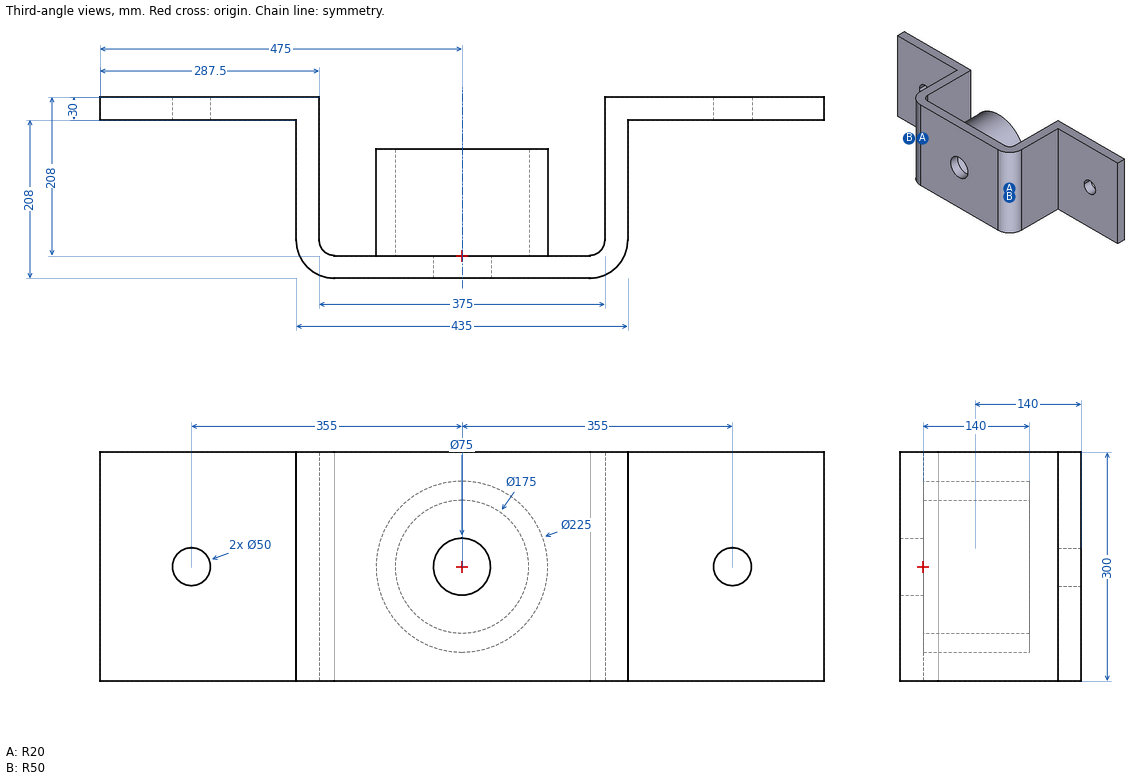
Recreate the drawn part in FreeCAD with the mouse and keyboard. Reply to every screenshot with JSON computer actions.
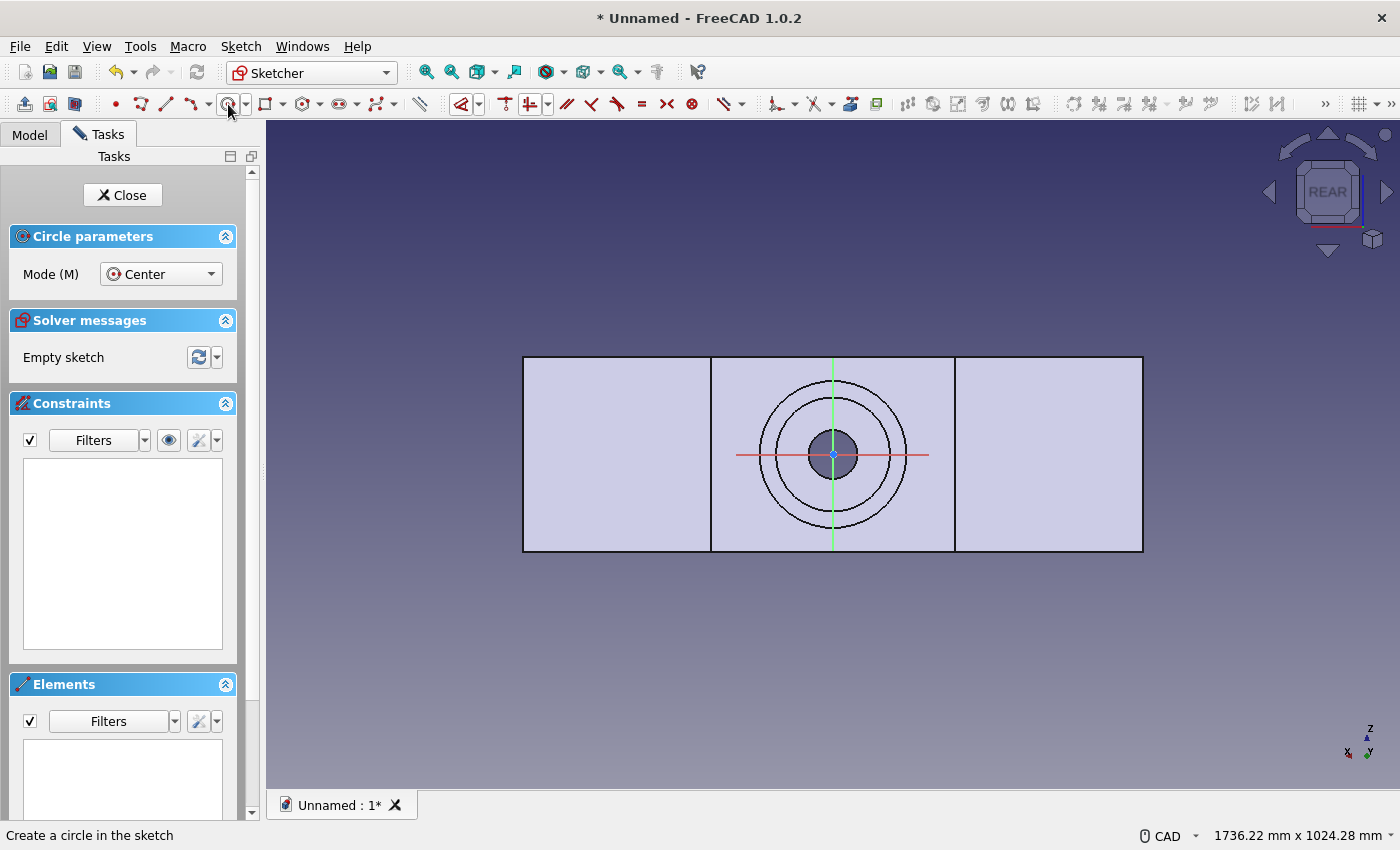
{"action": "scroll", "coordinate": [1065, 455], "scroll_direction": "up", "scroll_amount": 2}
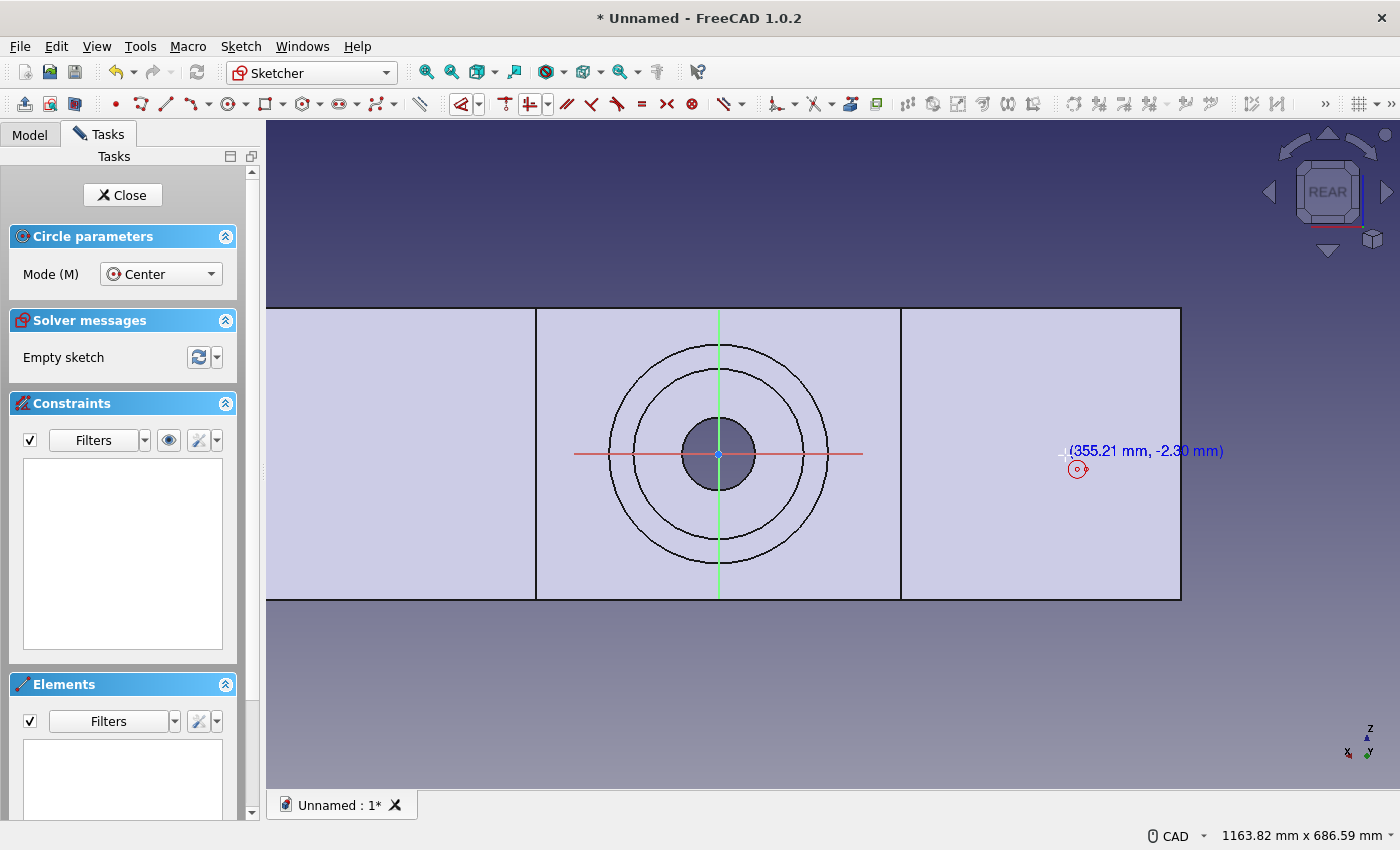
{"action": "left_click", "coordinate": [1064, 454]}
{"action": "mouse_move", "coordinate": [1082, 437]}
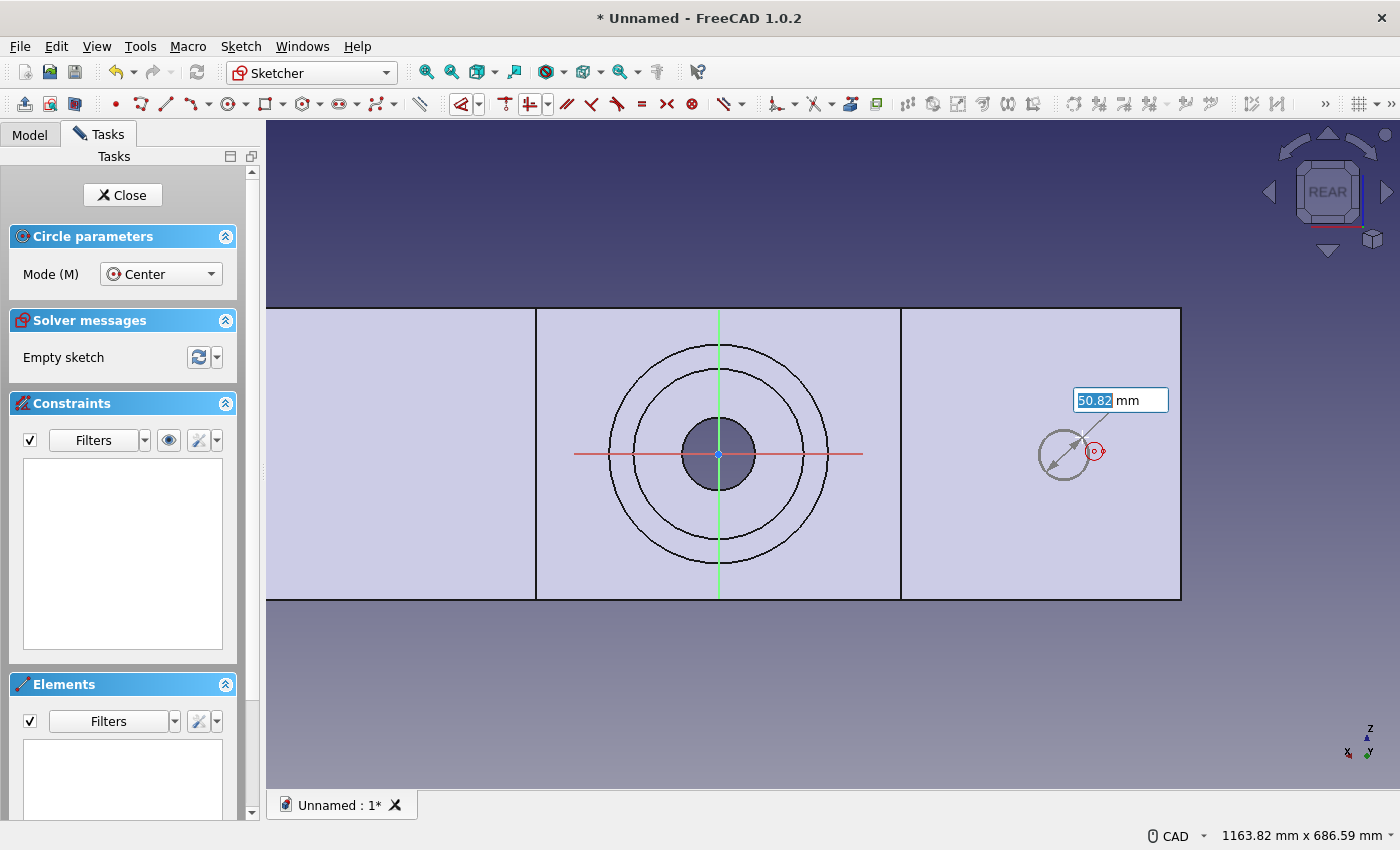
{"action": "type", "text": "50"}
{"action": "key", "text": "Return"}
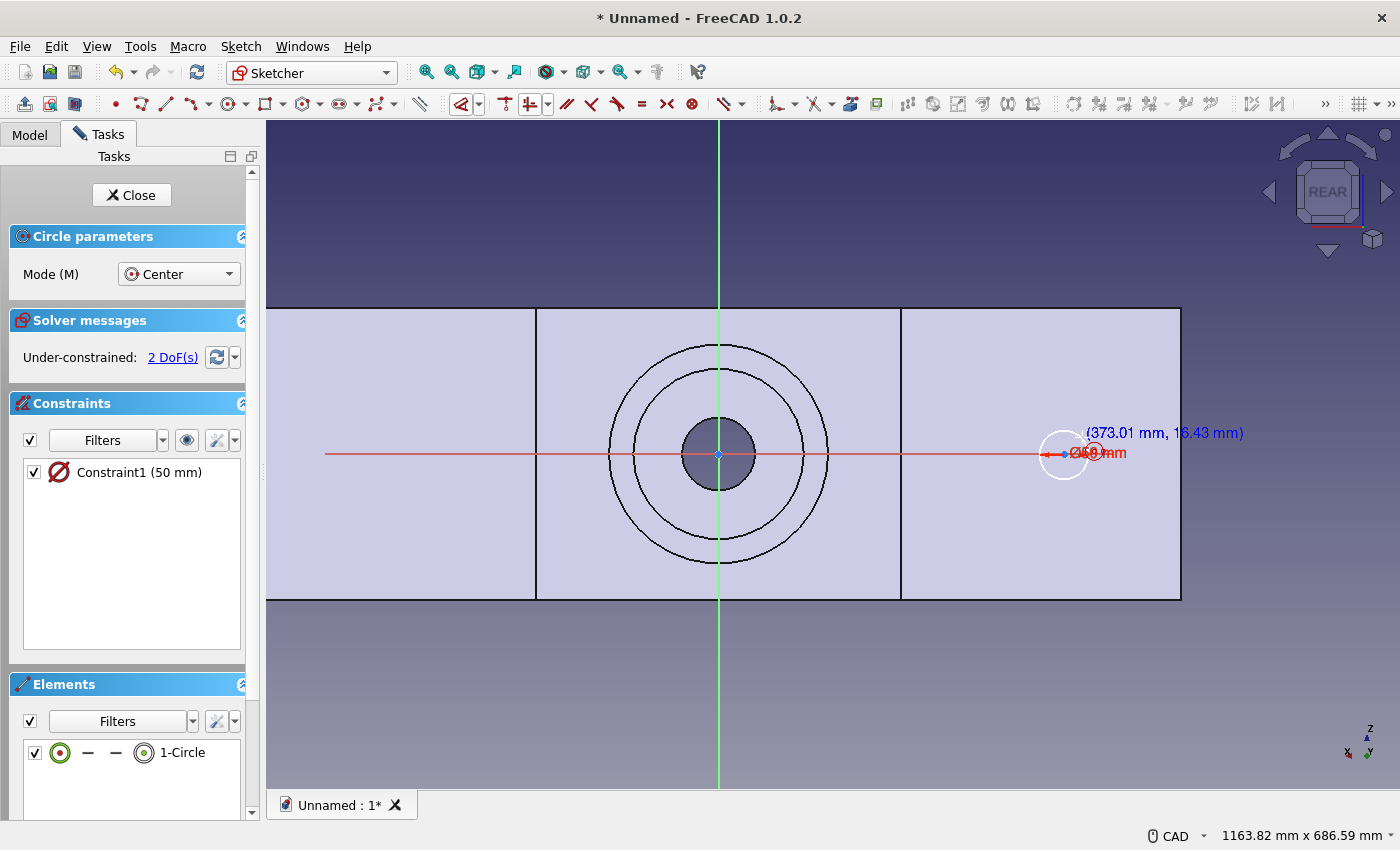
{"action": "left_click", "coordinate": [373, 454]}
{"action": "mouse_move", "coordinate": [390, 437]}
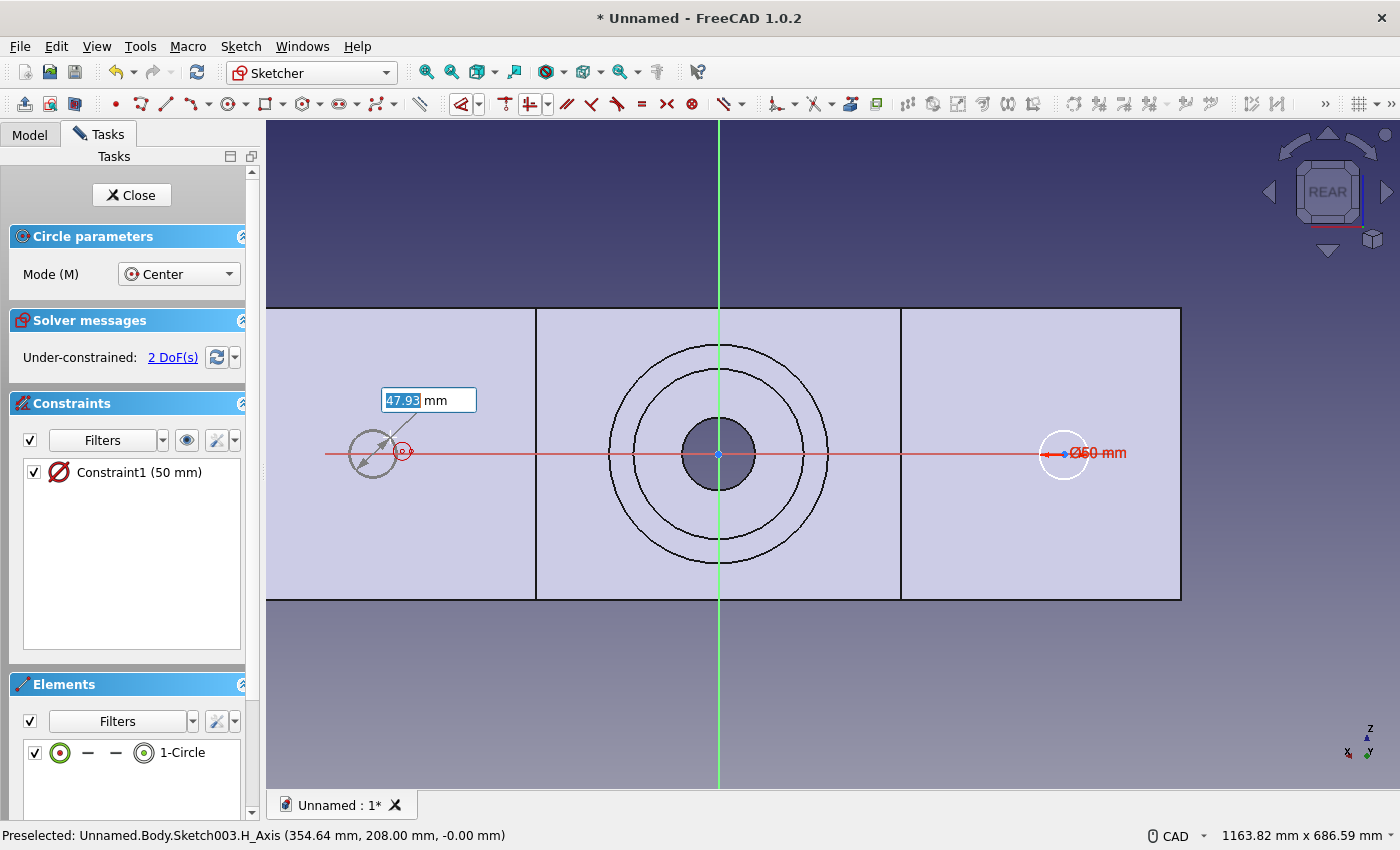
{"action": "type", "text": "50"}
{"action": "key", "text": "Return"}
{"action": "key", "text": "Escape"}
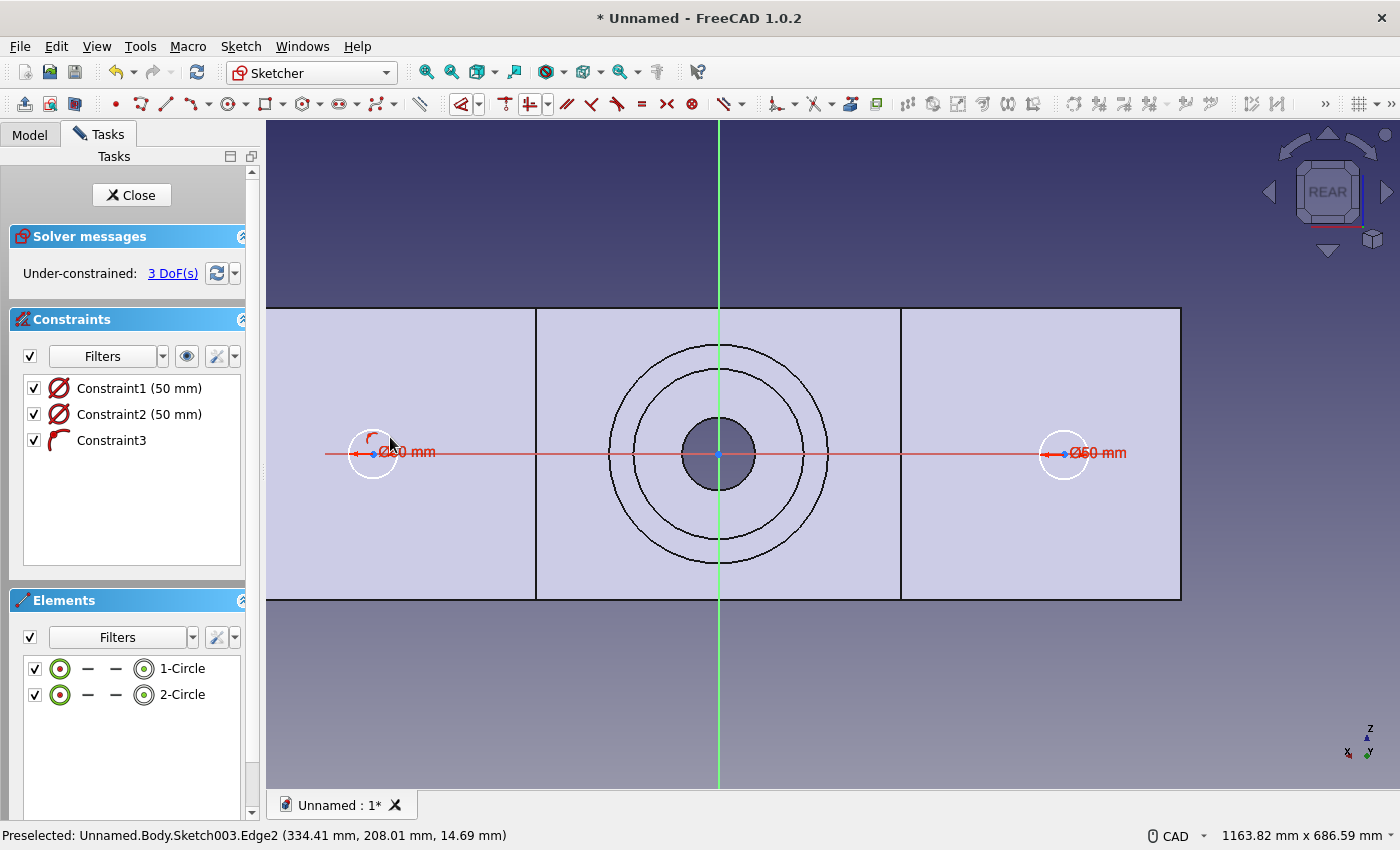
{"action": "left_click", "coordinate": [1064, 455]}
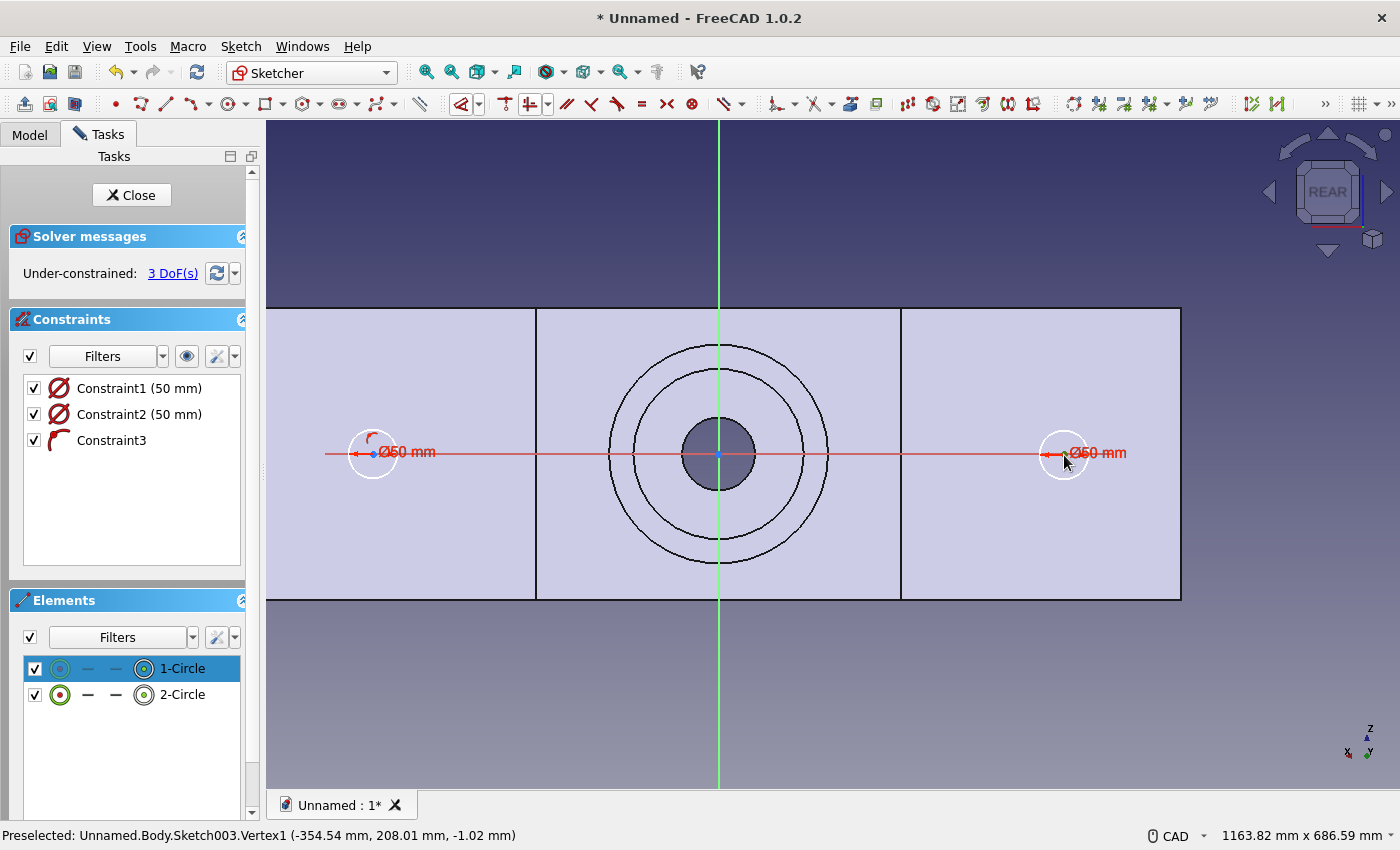
{"action": "left_click", "coordinate": [496, 454]}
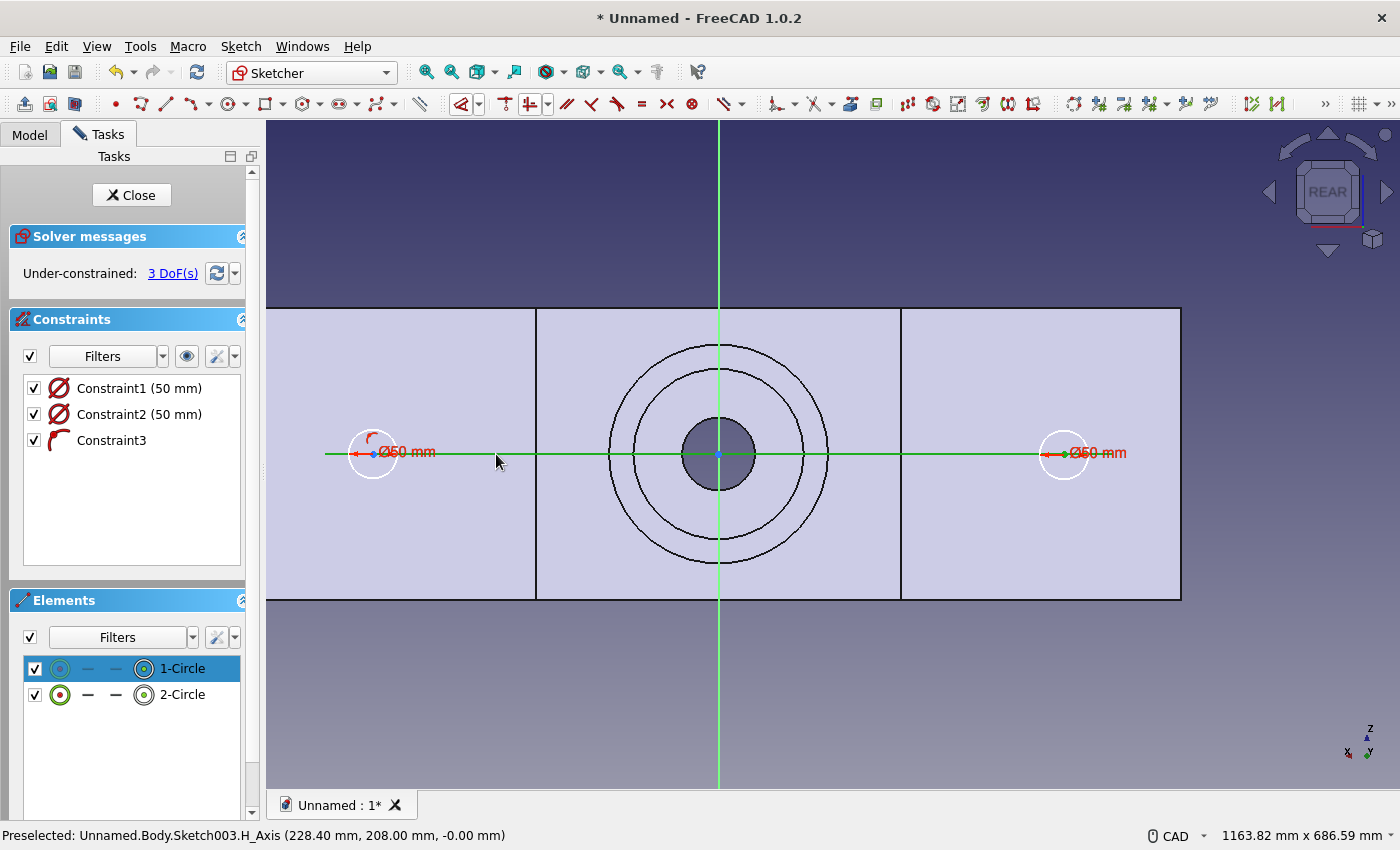
{"action": "left_click", "coordinate": [505, 104]}